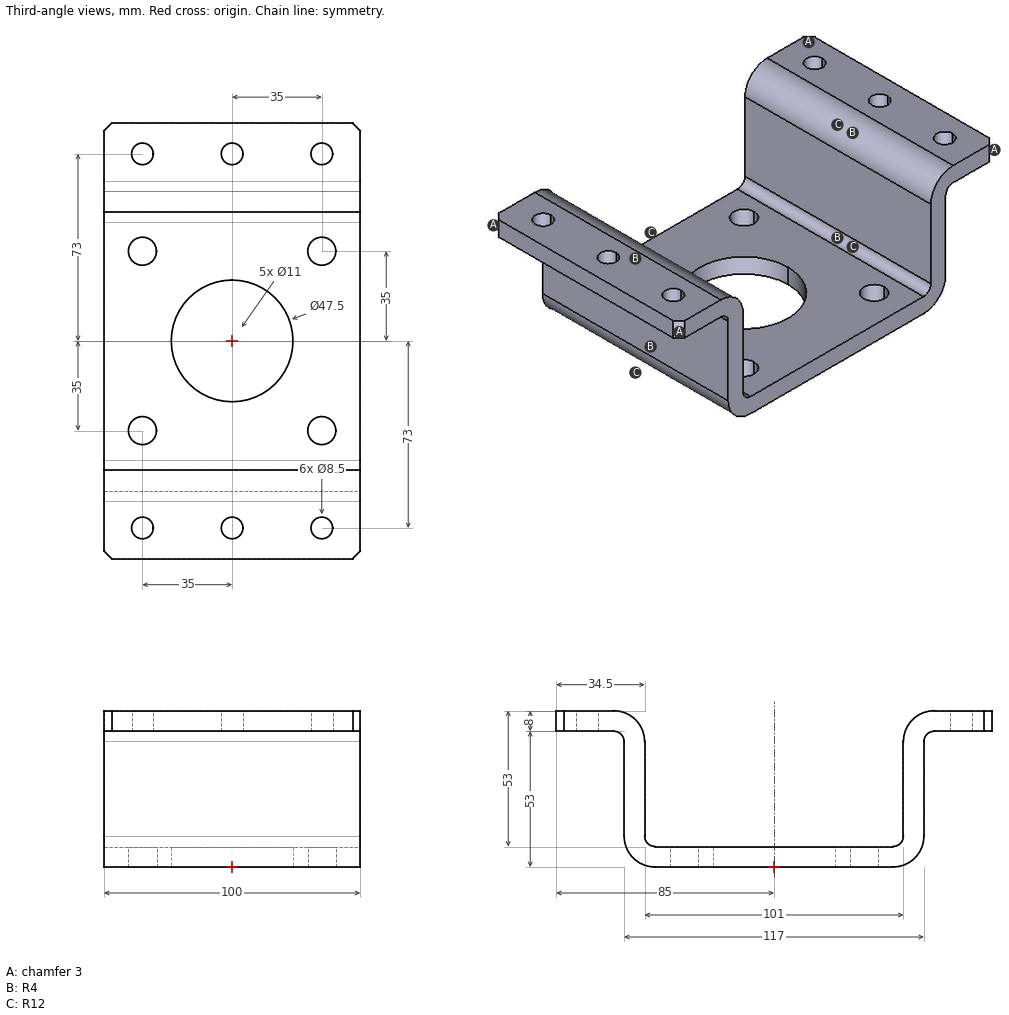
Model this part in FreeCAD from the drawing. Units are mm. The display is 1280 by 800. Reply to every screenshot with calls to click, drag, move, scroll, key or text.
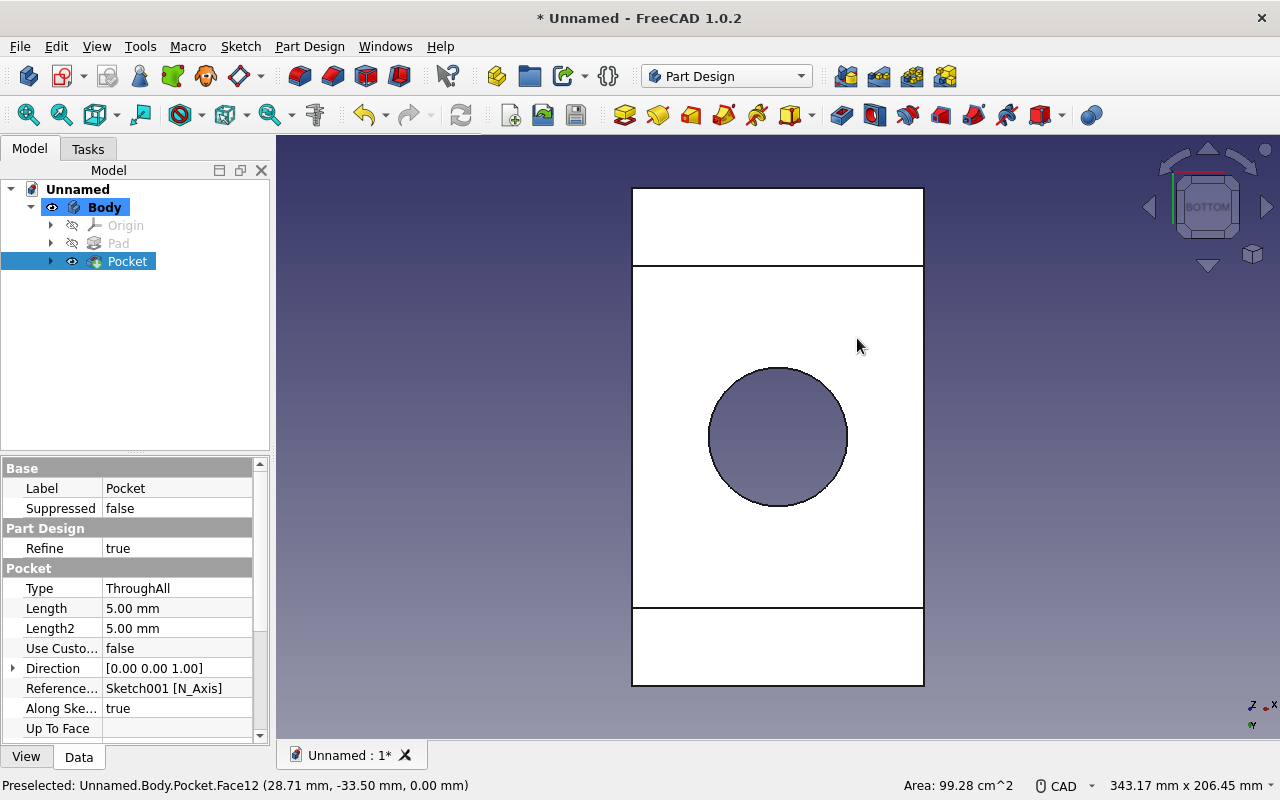
click(62, 76)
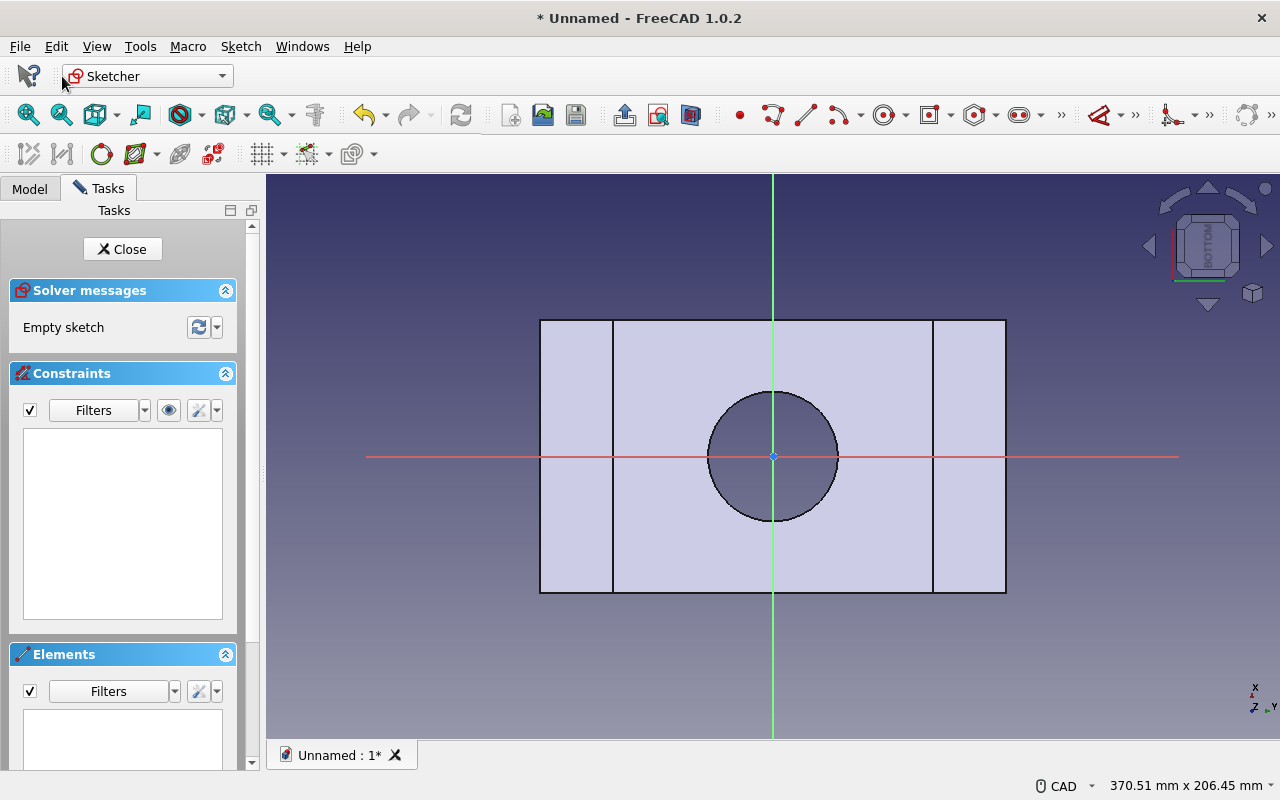
scroll(912, 456, up, 2)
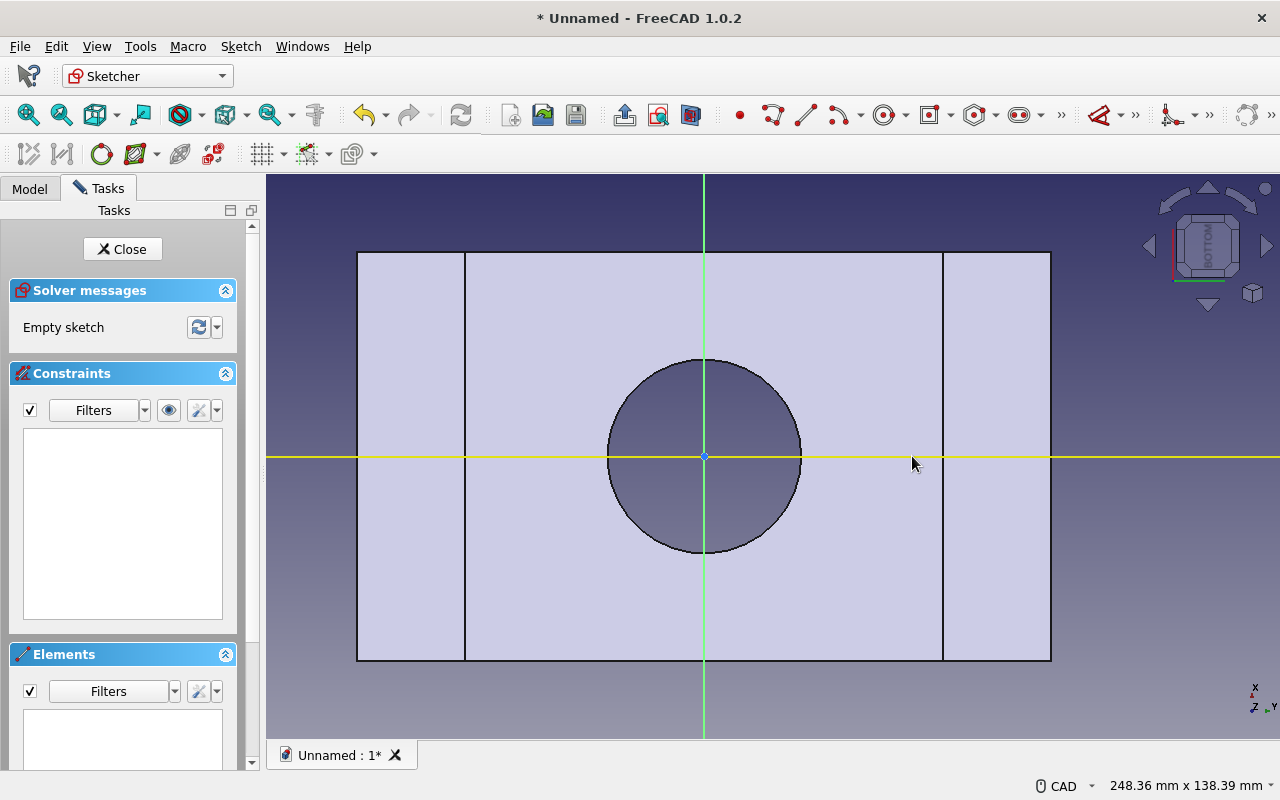
key(g)
key(c)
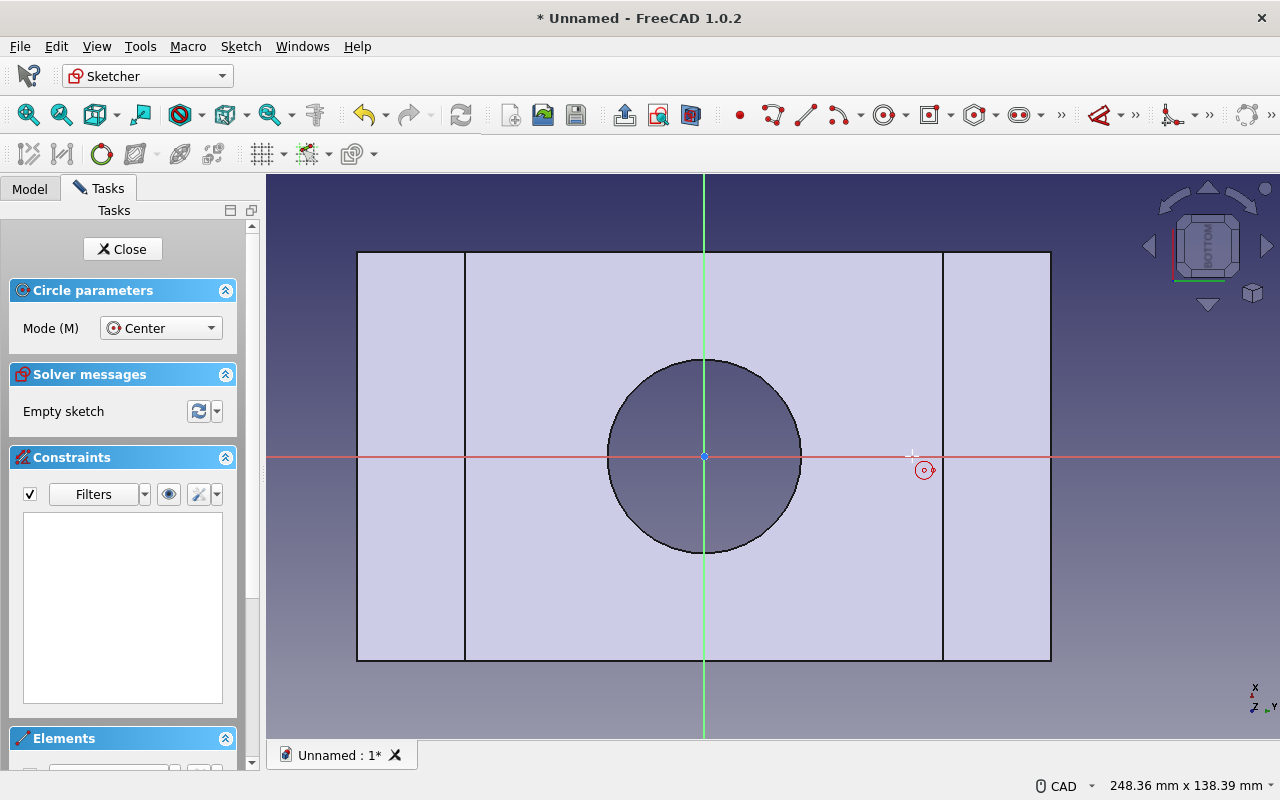
click(704, 456)
move(720, 441)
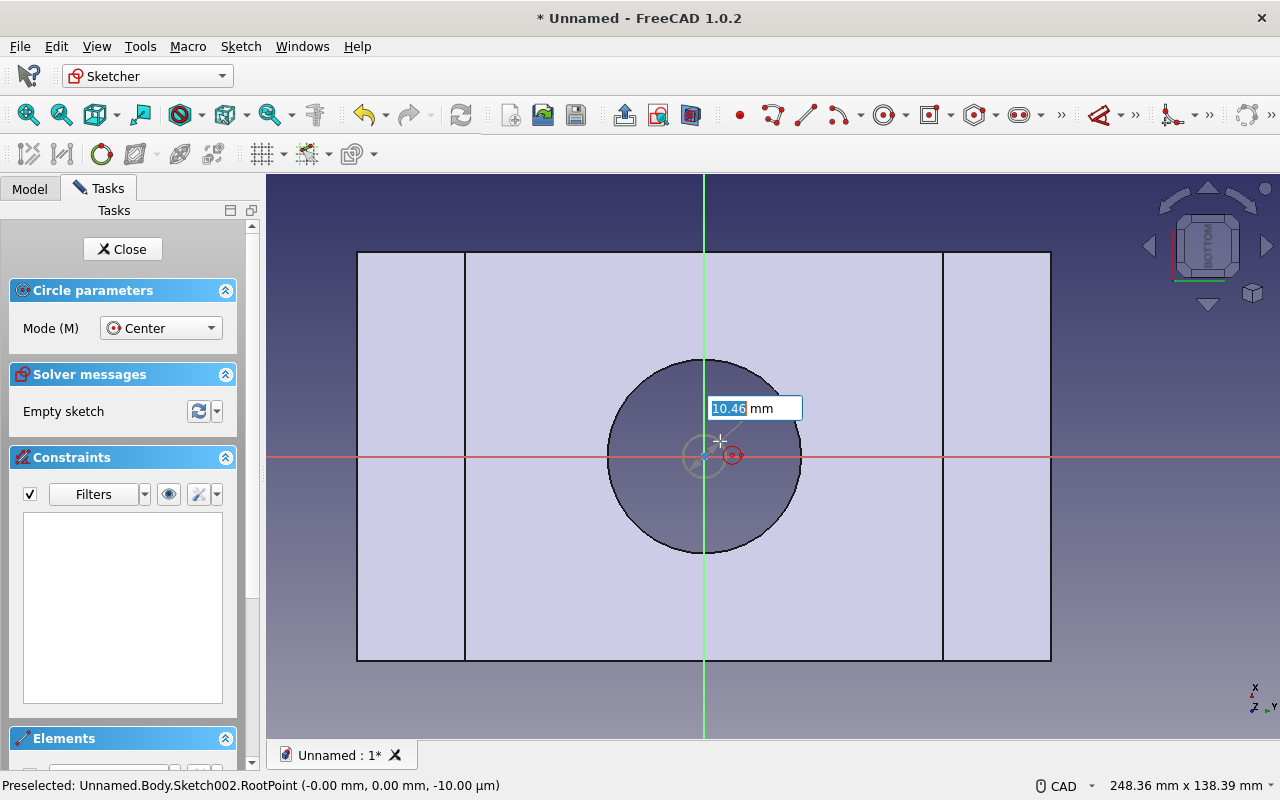
text(11)
key(Return)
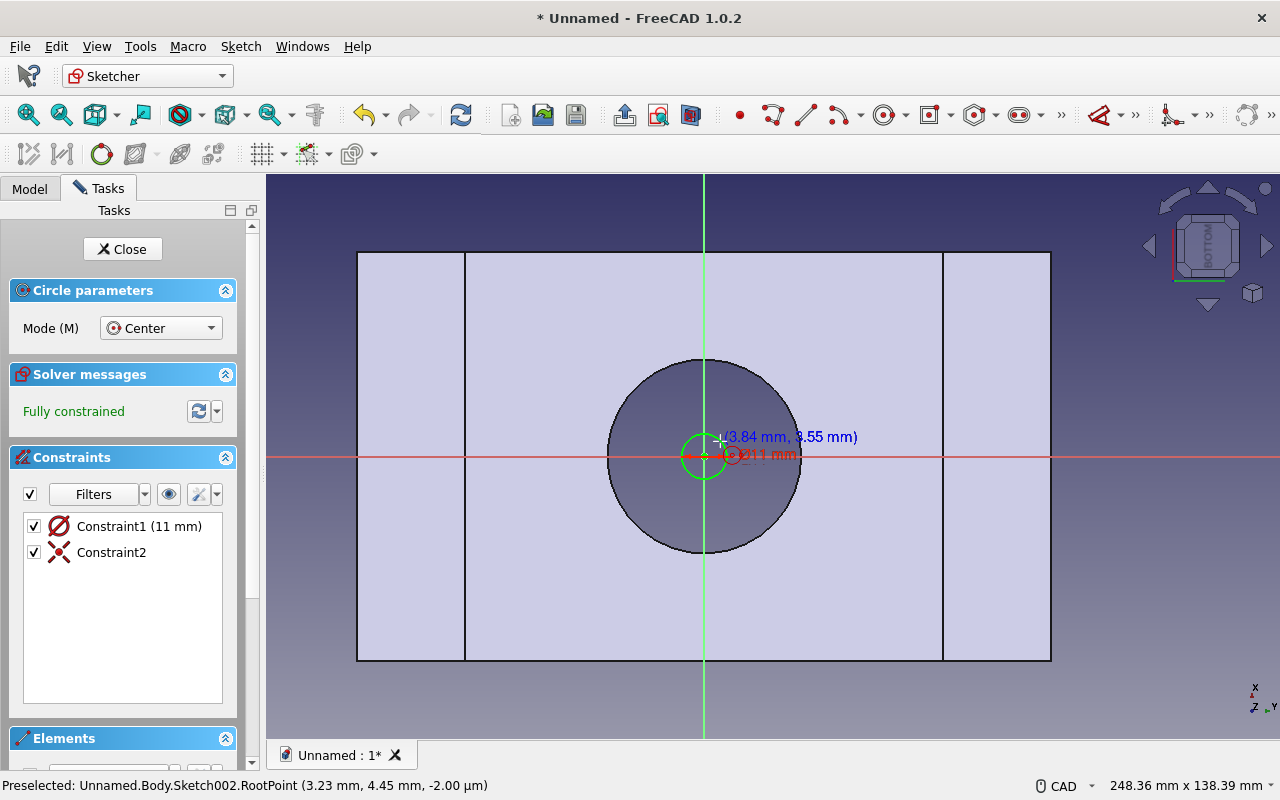
click(561, 599)
move(577, 584)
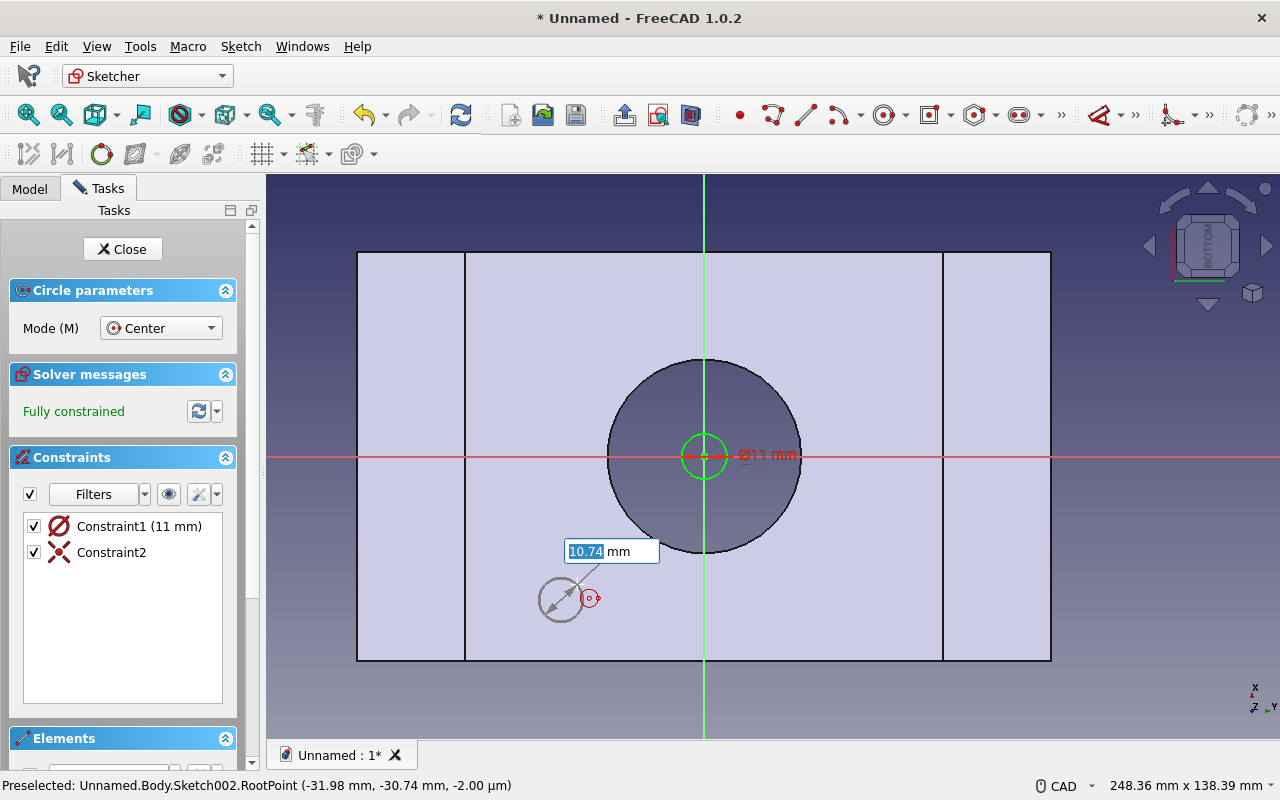
text(11)
key(Return)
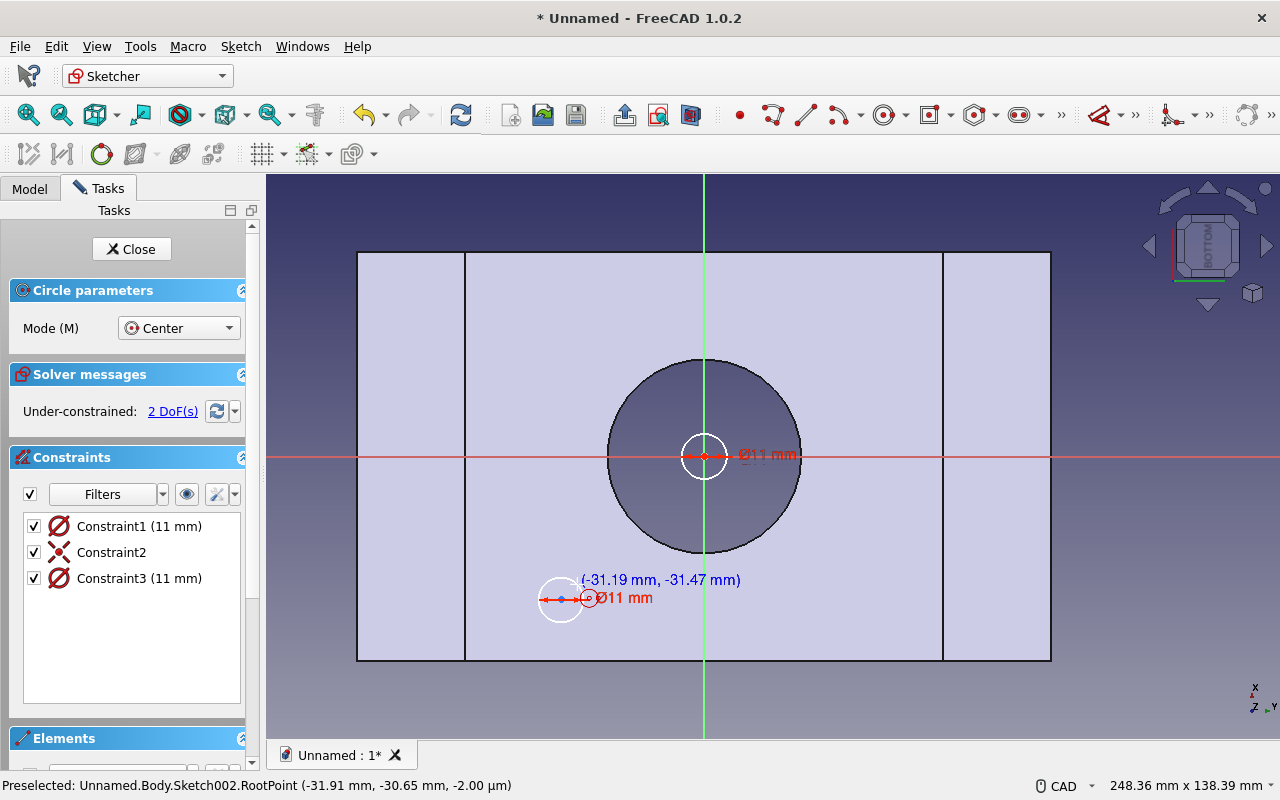
click(847, 314)
move(863, 298)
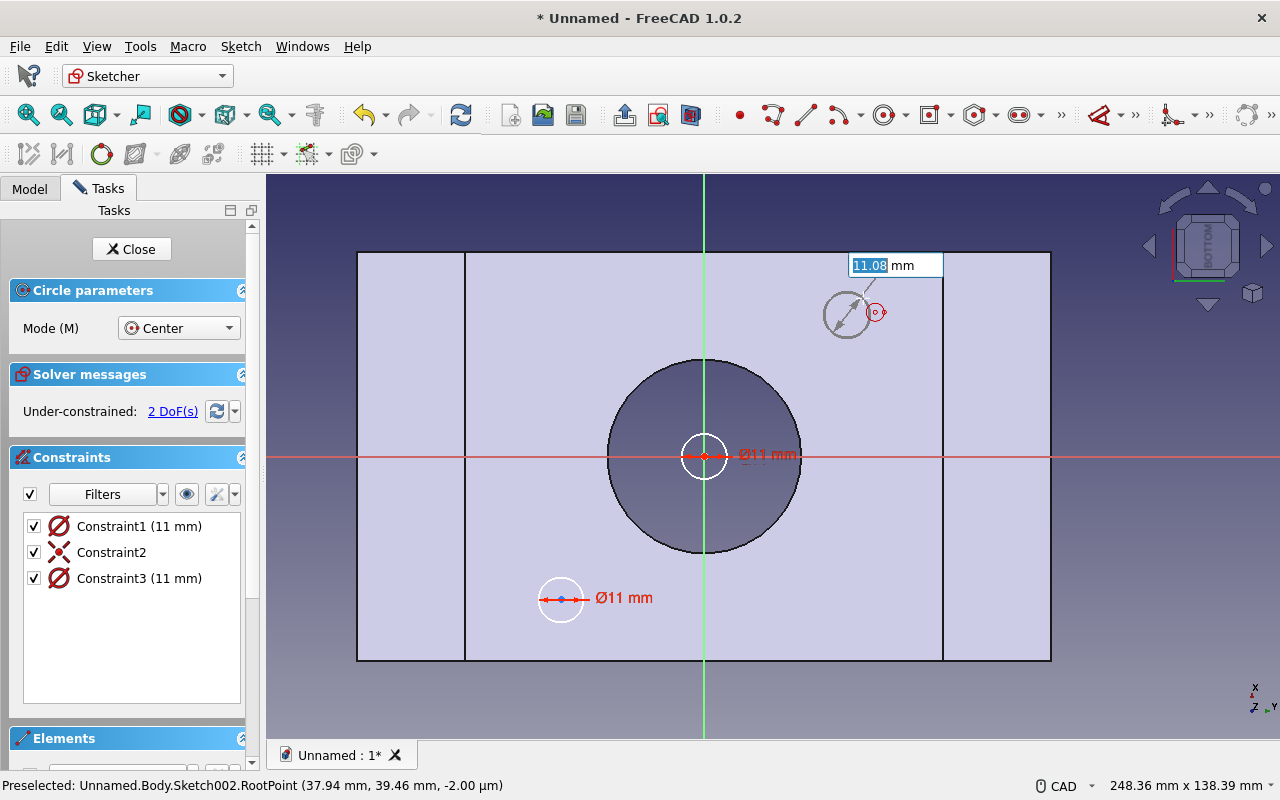
text(11)
key(Return)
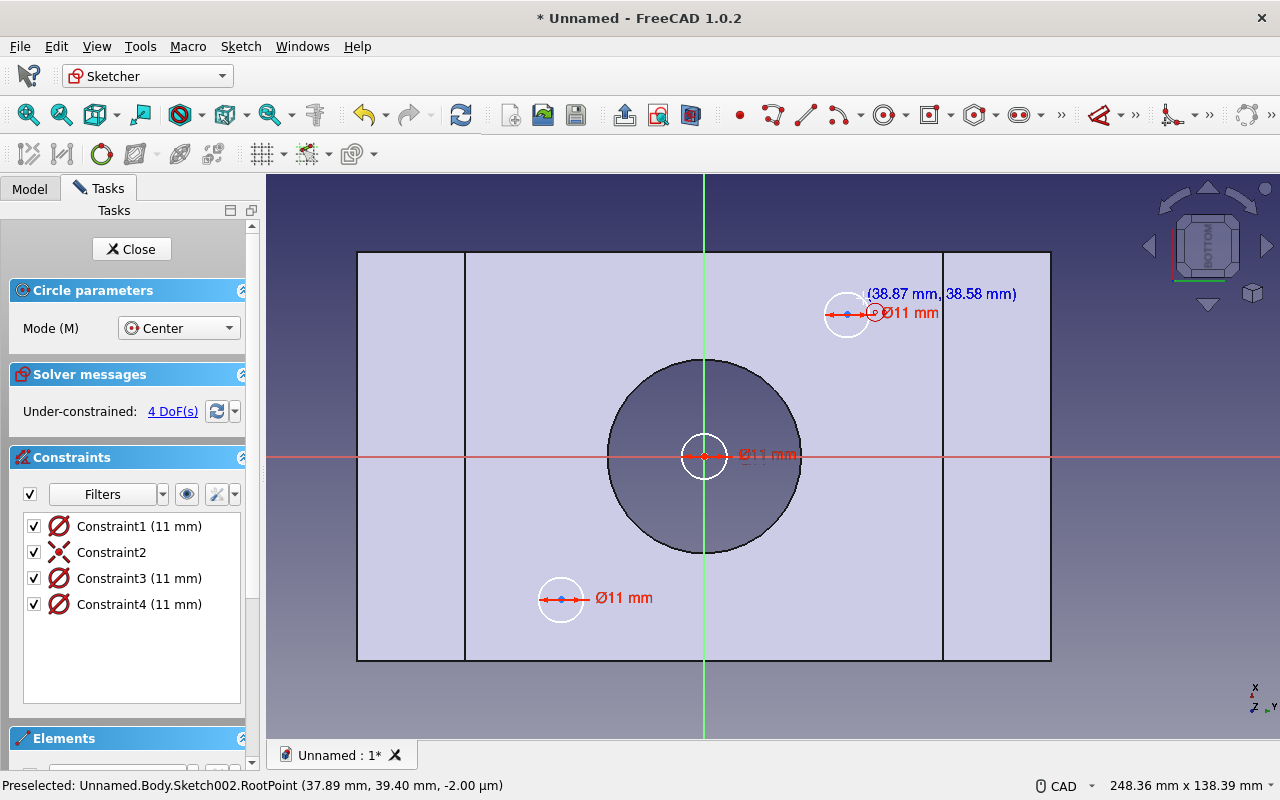
click(561, 314)
move(577, 298)